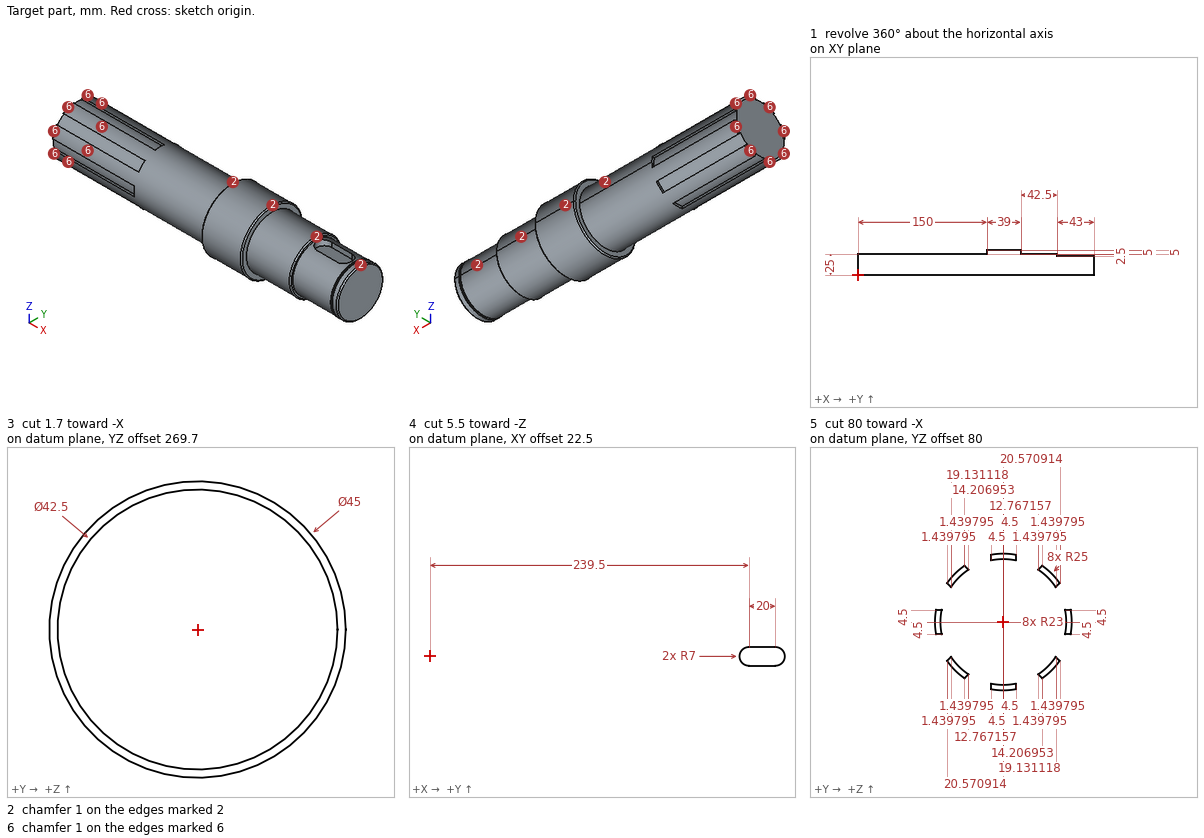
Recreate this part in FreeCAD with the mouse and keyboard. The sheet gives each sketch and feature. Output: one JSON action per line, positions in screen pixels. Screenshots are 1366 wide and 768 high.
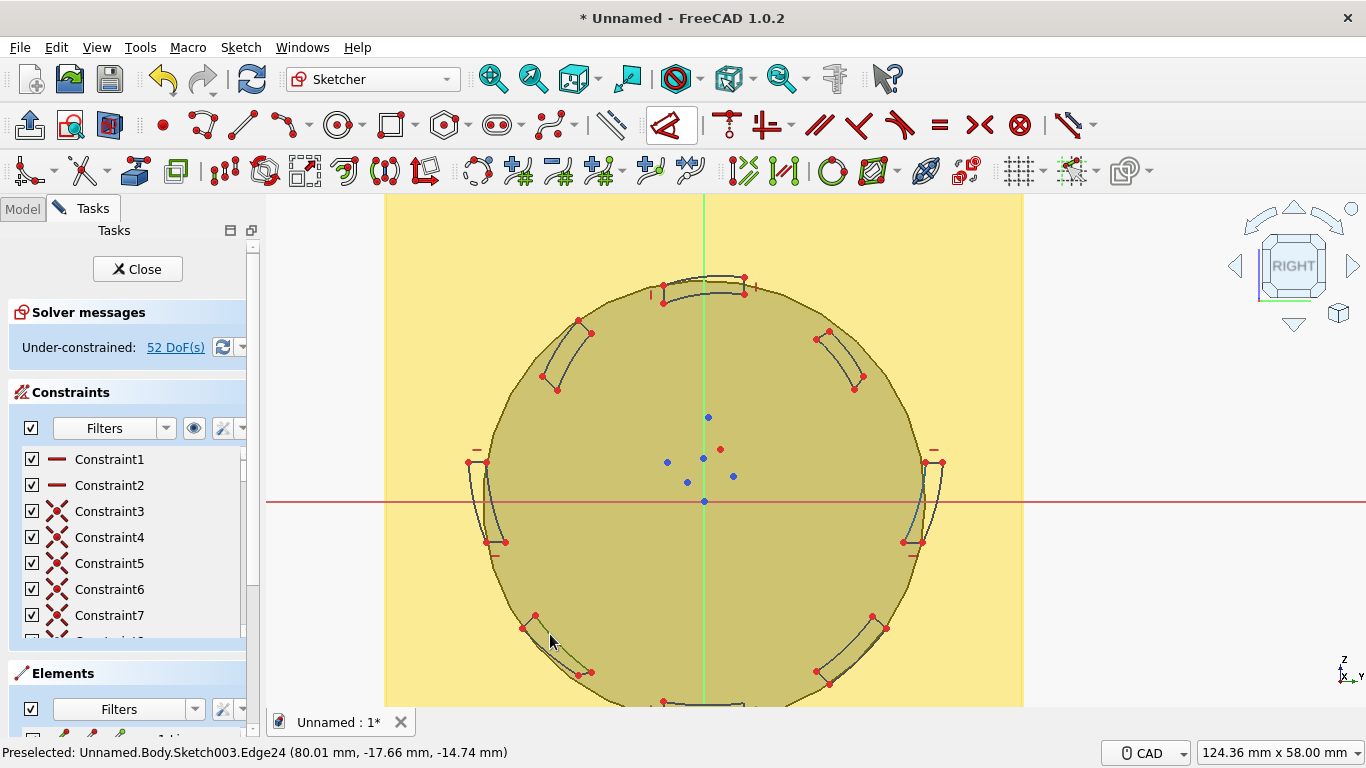
{"action": "left_click", "coordinate": [728, 126]}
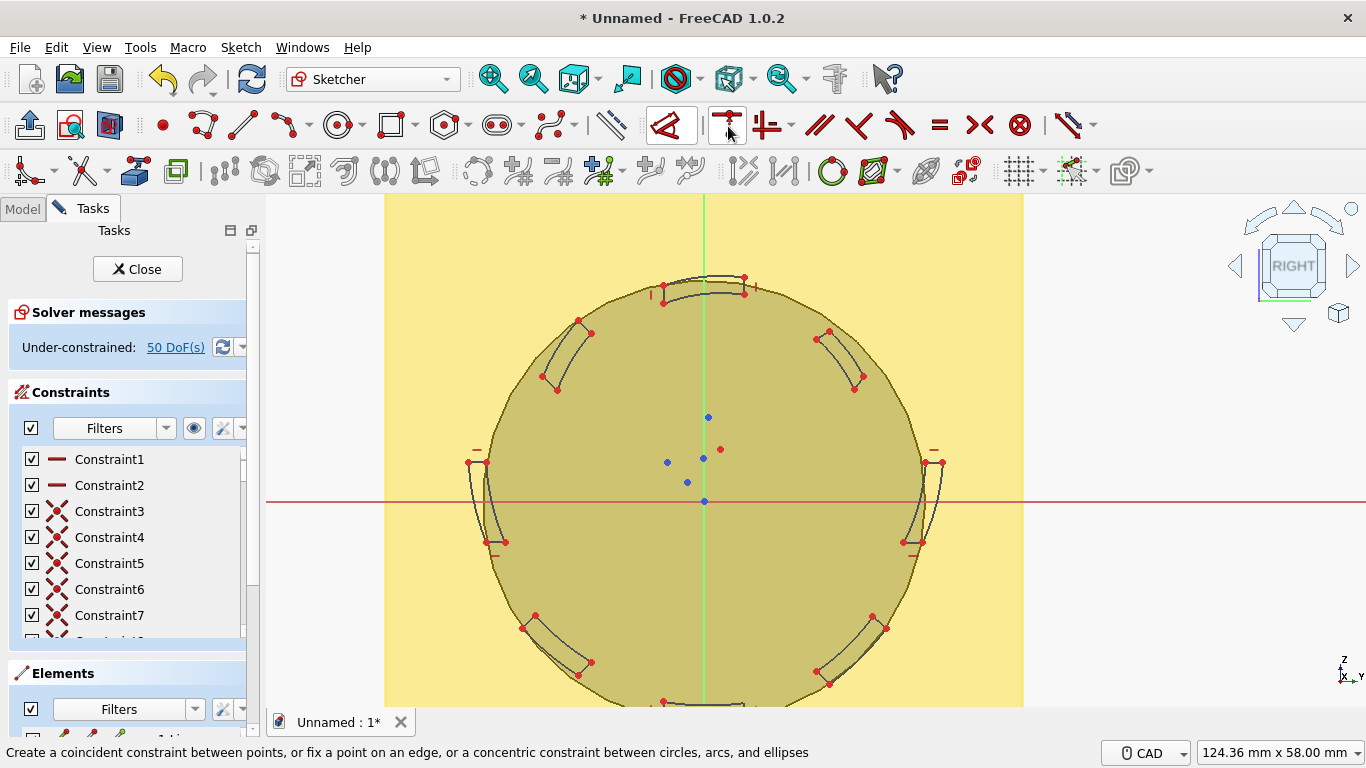
{"action": "left_click", "coordinate": [914, 520]}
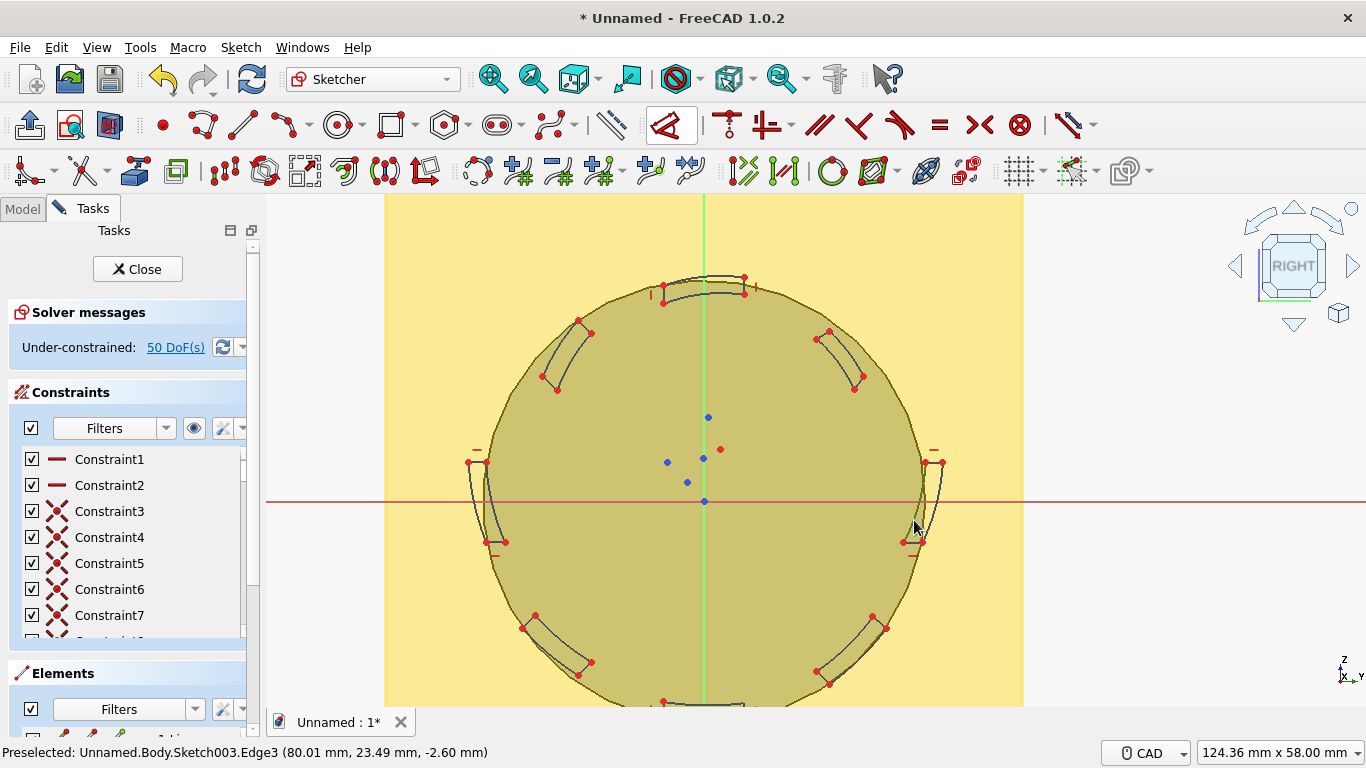
{"action": "scroll", "coordinate": [836, 347], "scroll_direction": "down", "scroll_amount": 2}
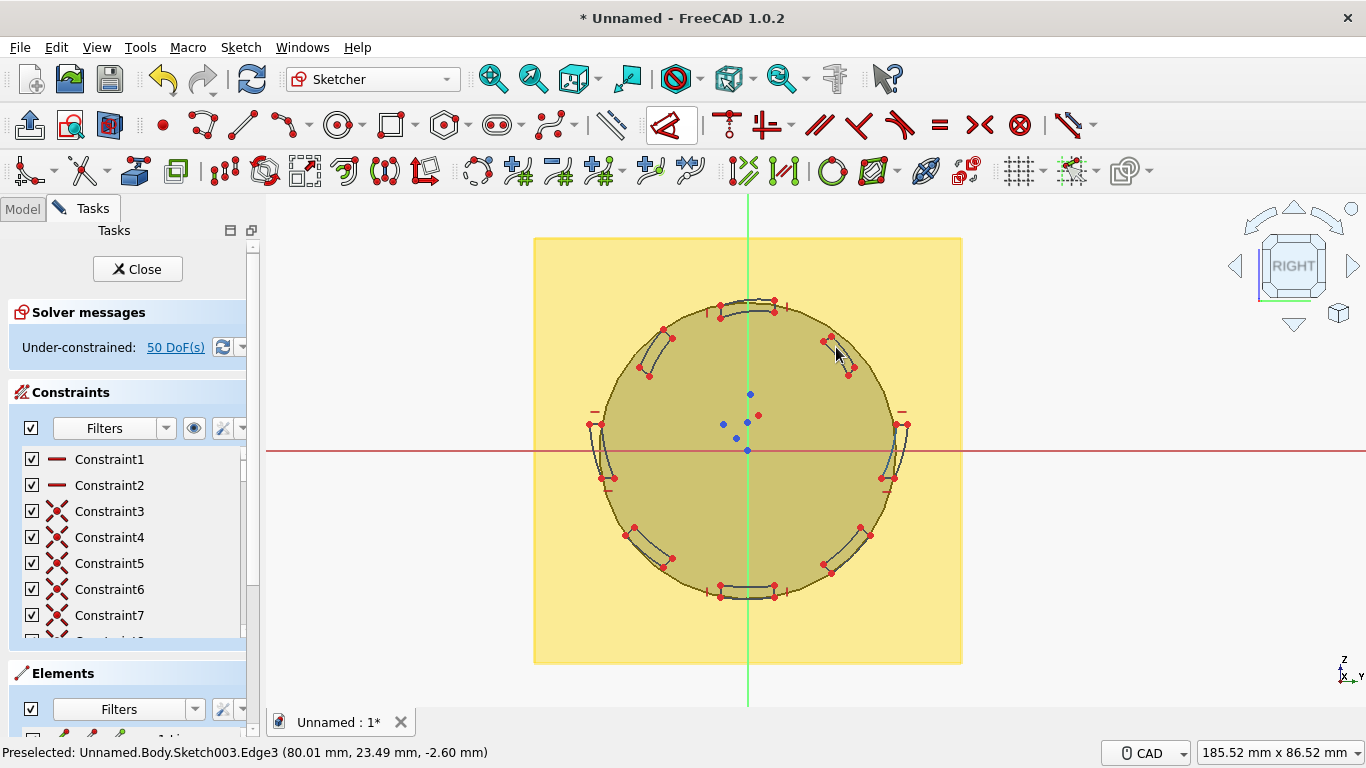
{"action": "scroll", "coordinate": [737, 599], "scroll_direction": "up", "scroll_amount": 2}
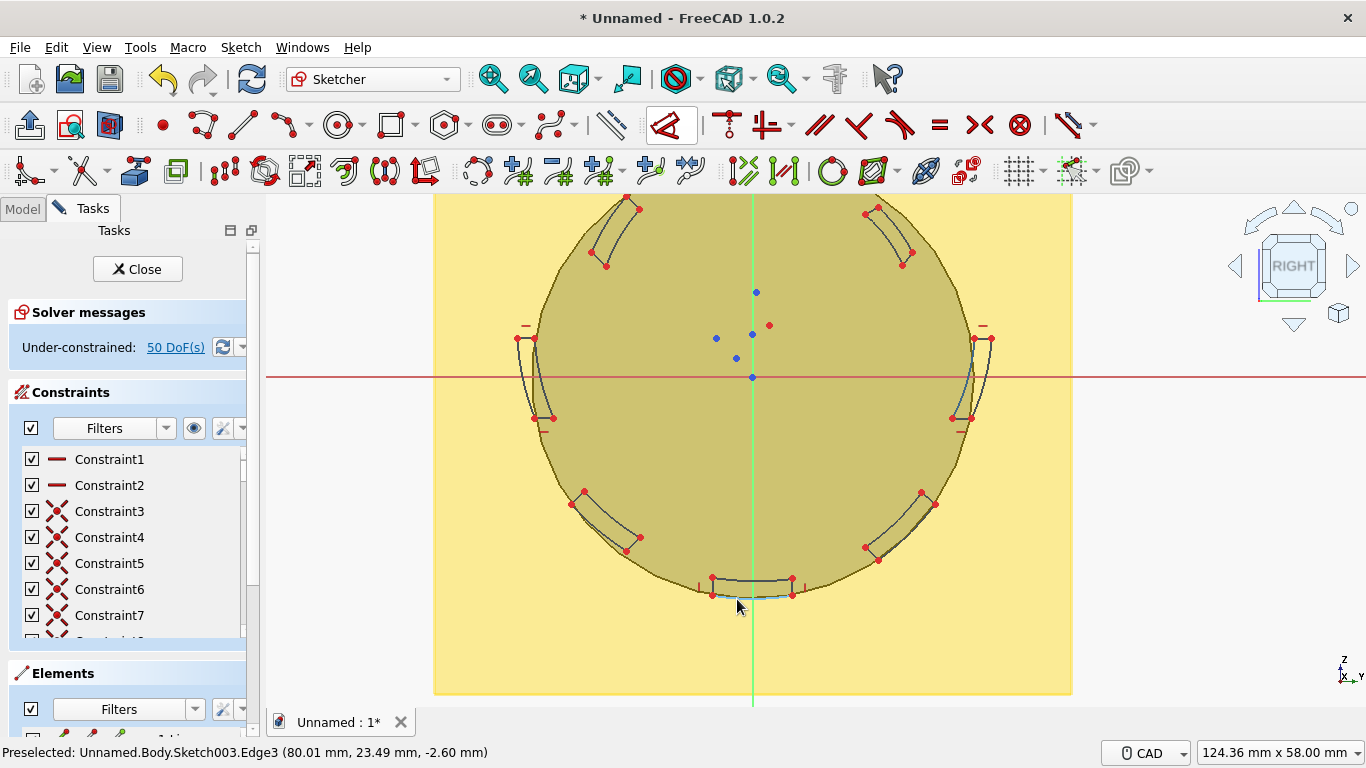
{"action": "left_click", "coordinate": [736, 598]}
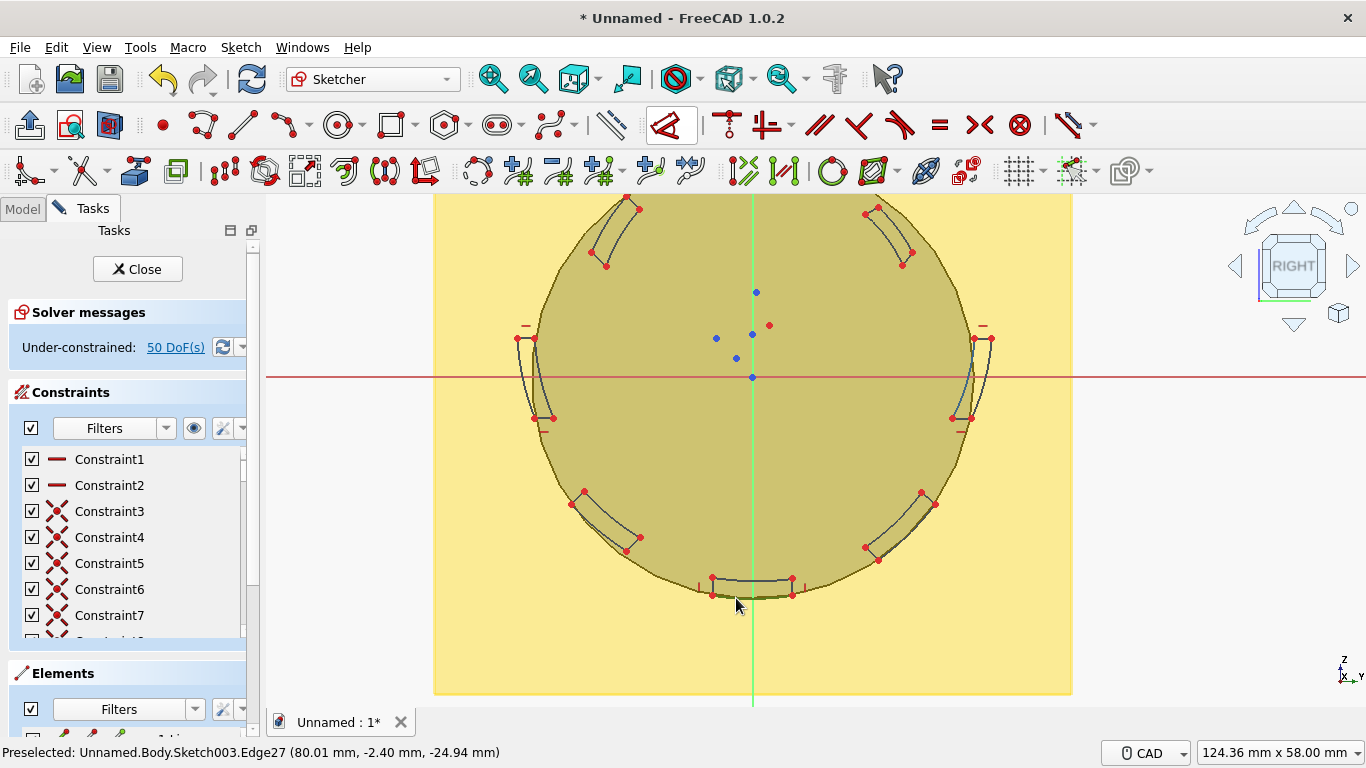
{"action": "left_click", "coordinate": [728, 126]}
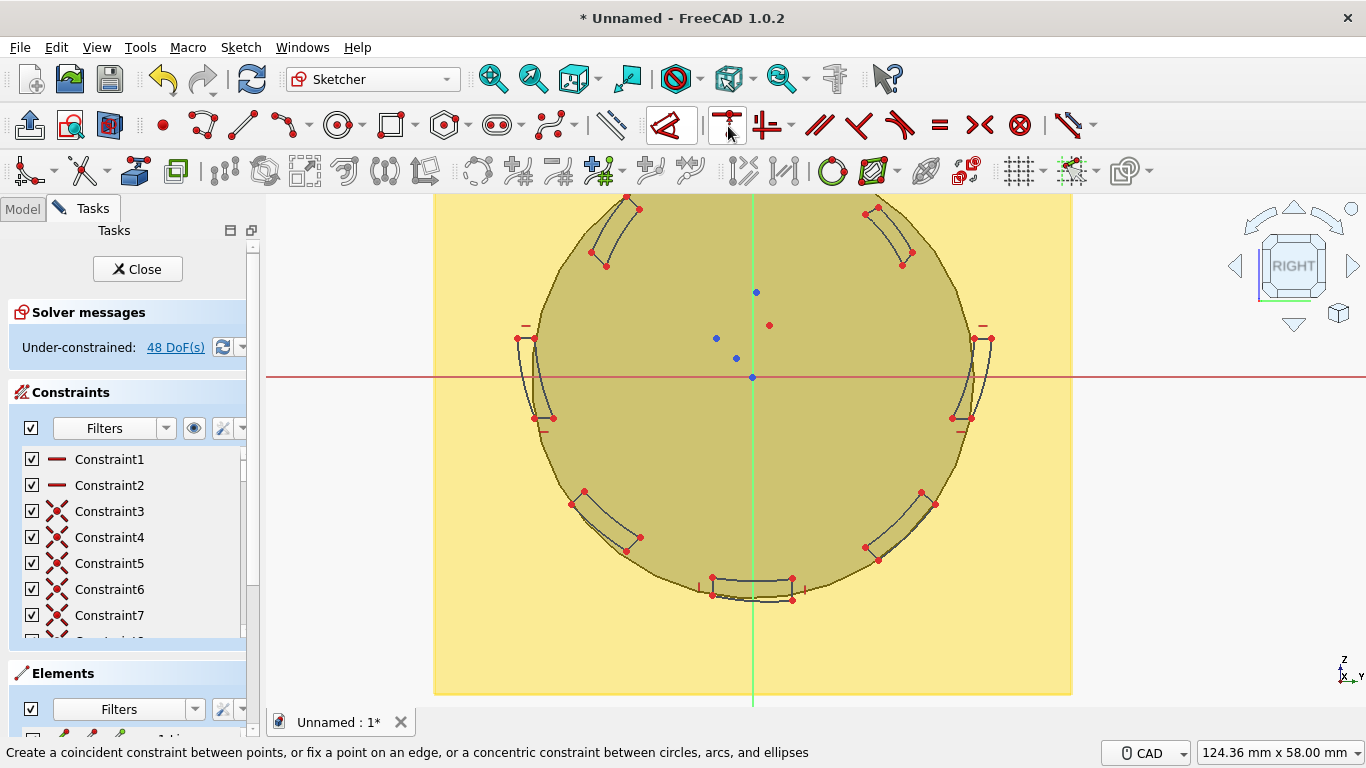
{"action": "left_click", "coordinate": [962, 396]}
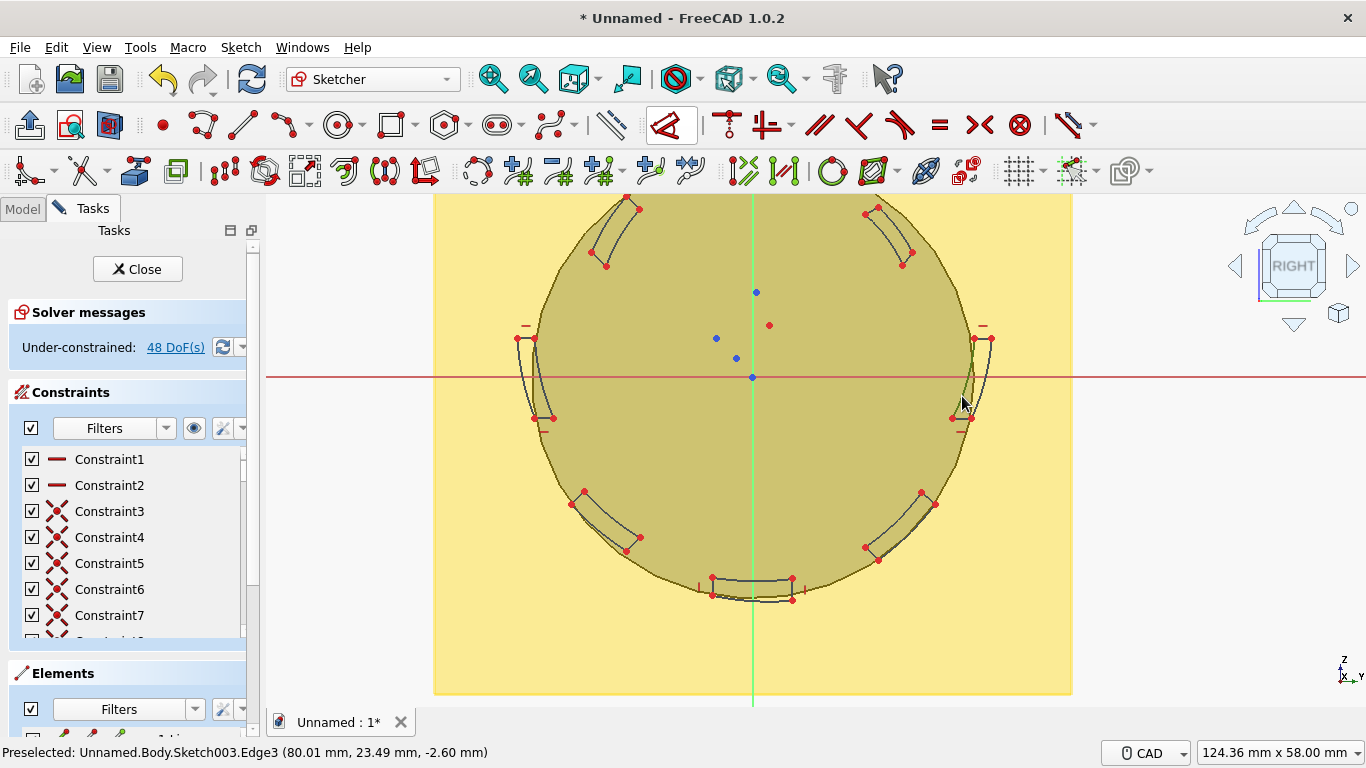
{"action": "left_click", "coordinate": [736, 580]}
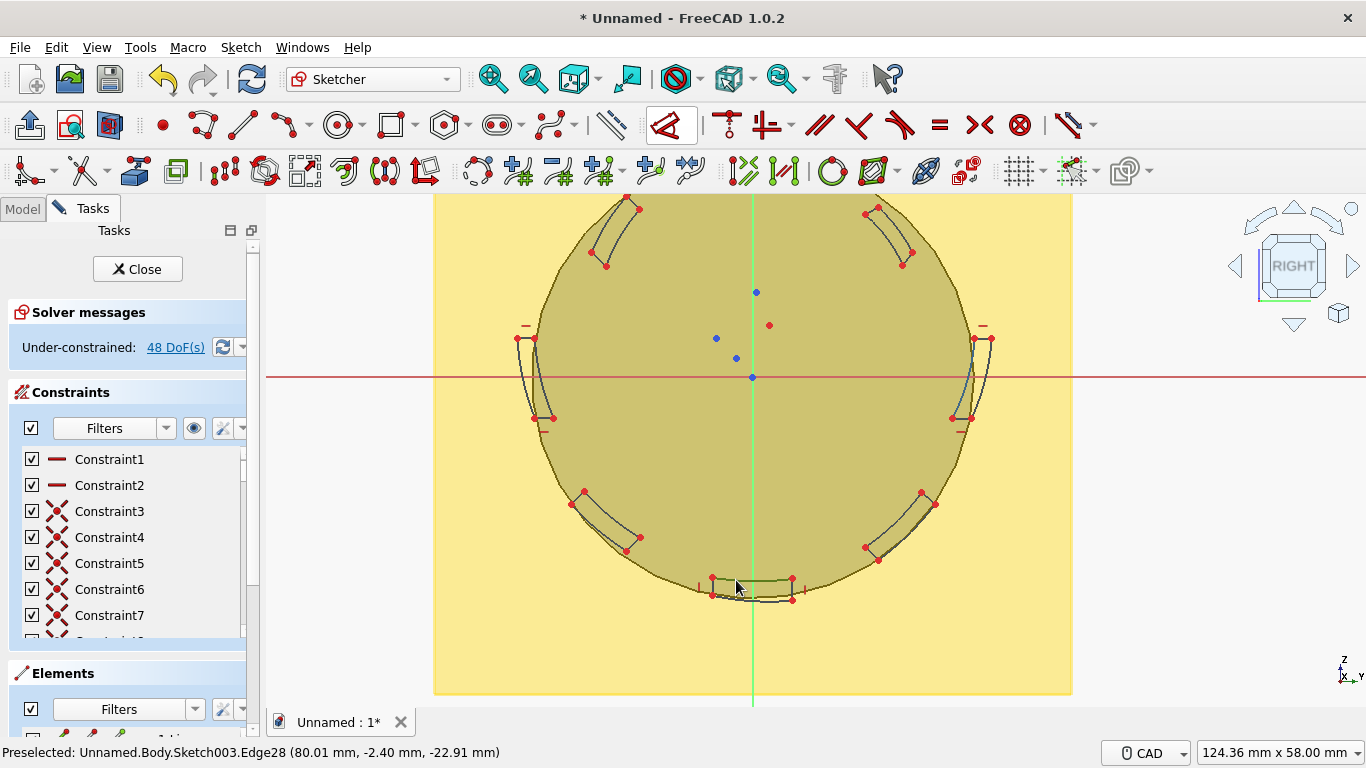
{"action": "left_click", "coordinate": [728, 126]}